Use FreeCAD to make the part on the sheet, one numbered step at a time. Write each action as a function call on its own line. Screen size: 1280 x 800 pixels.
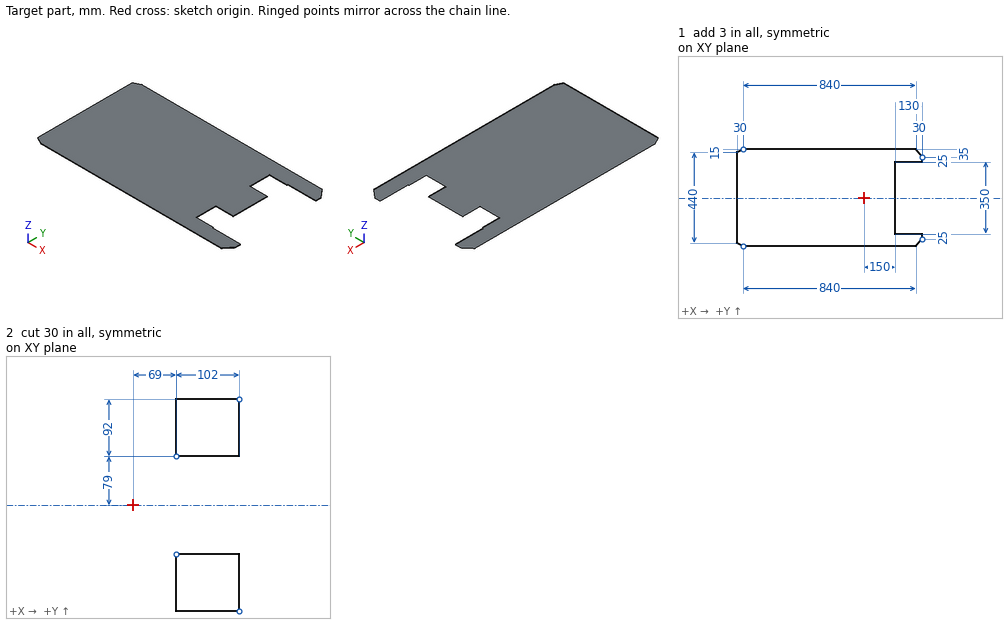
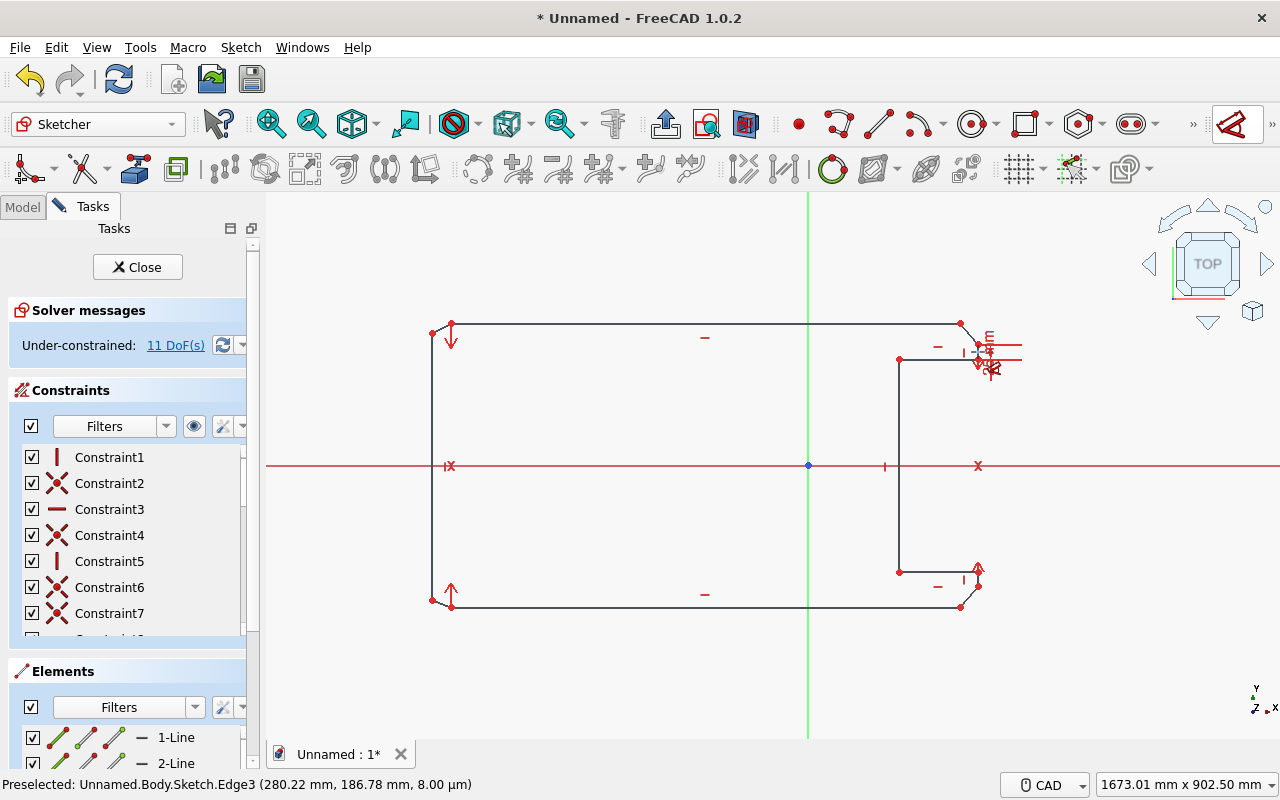
scroll(978, 583, up, 6)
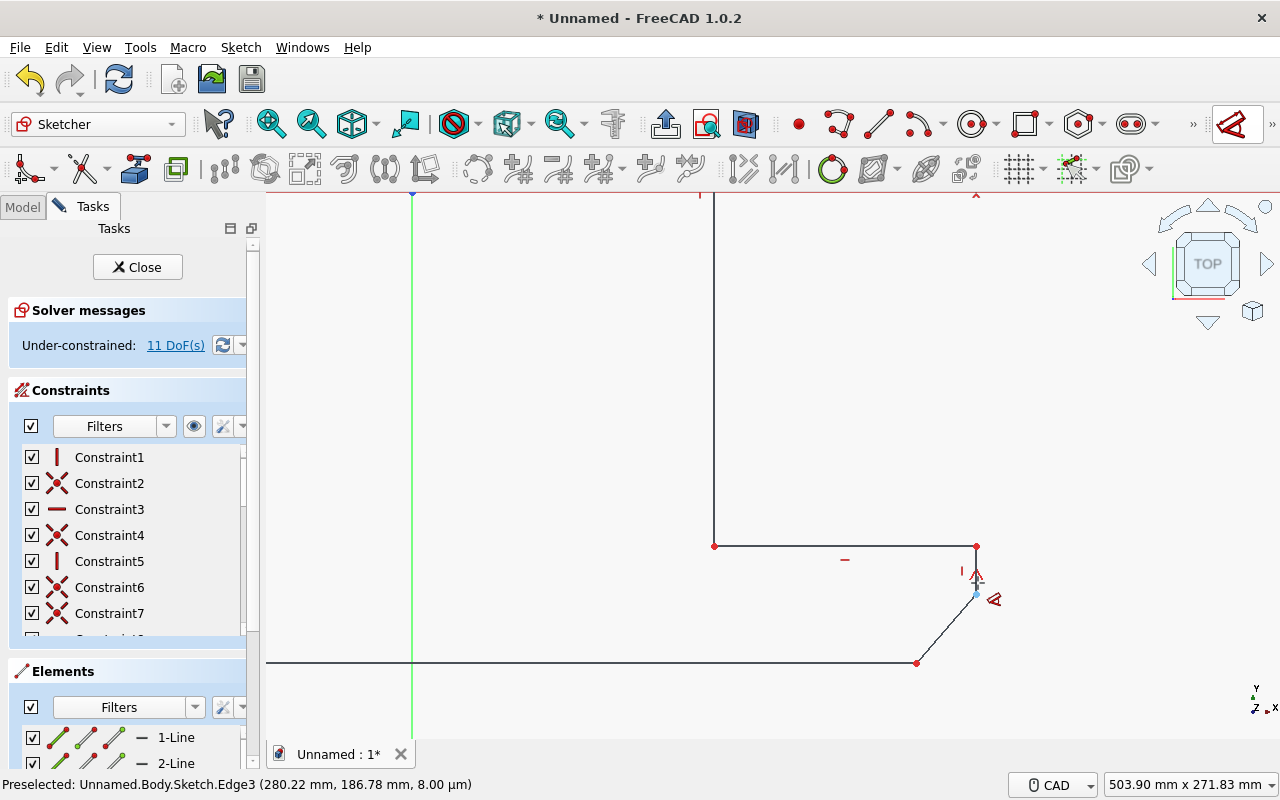
click(976, 580)
click(1010, 570)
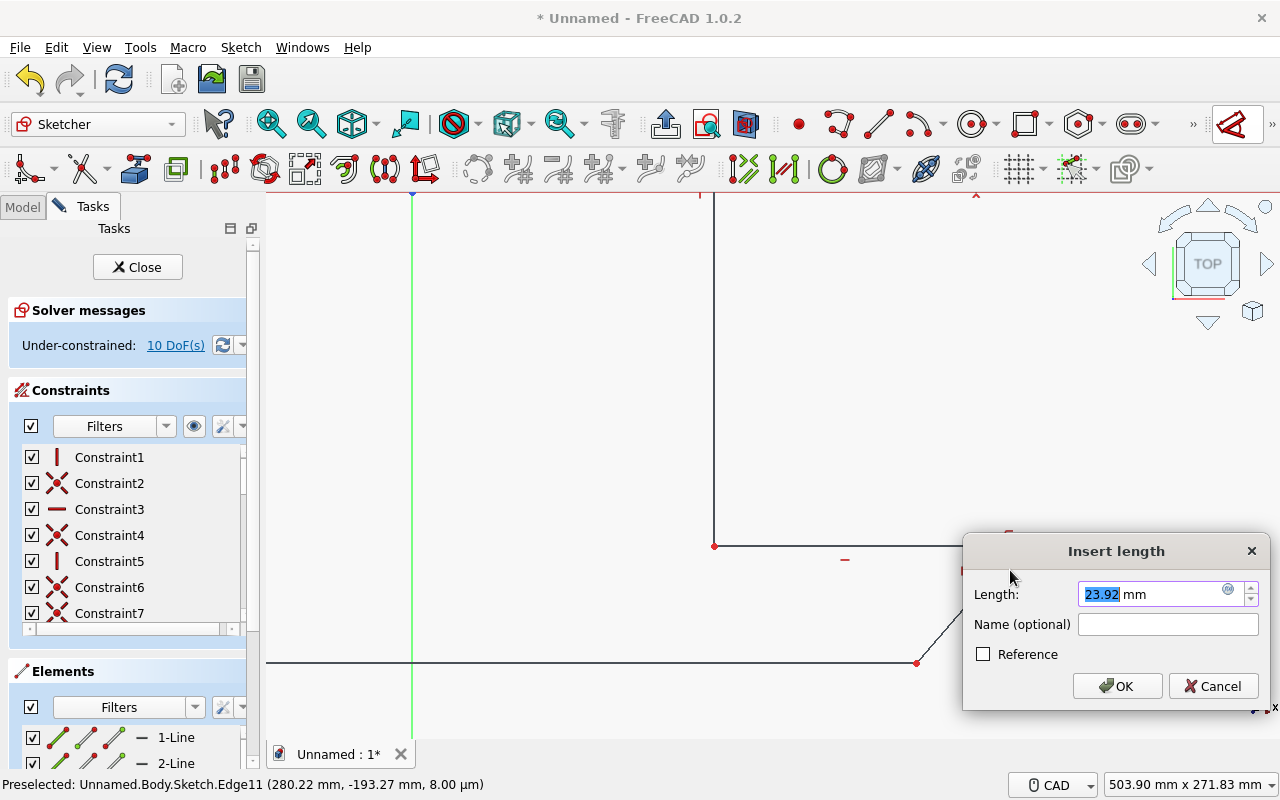
text(25)
key(Return)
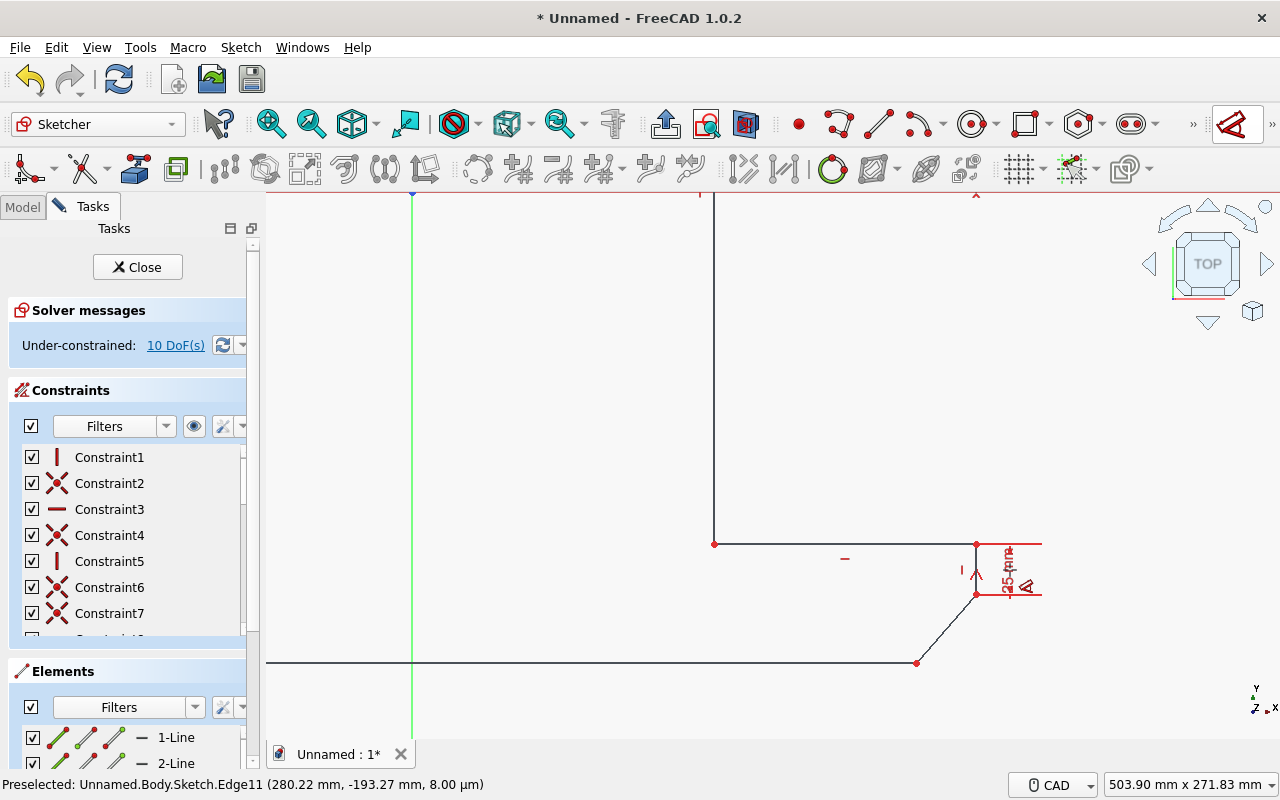
click(714, 333)
click(748, 382)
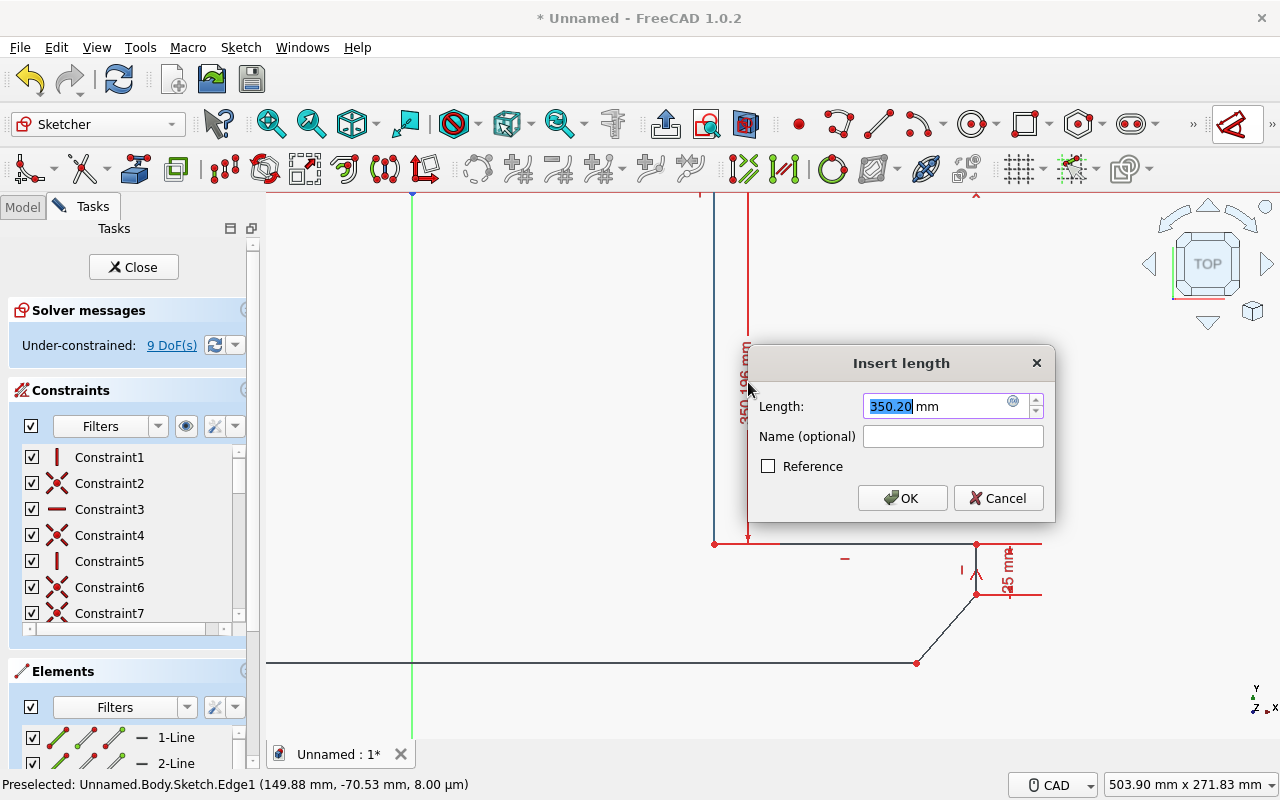
text(350)
key(Return)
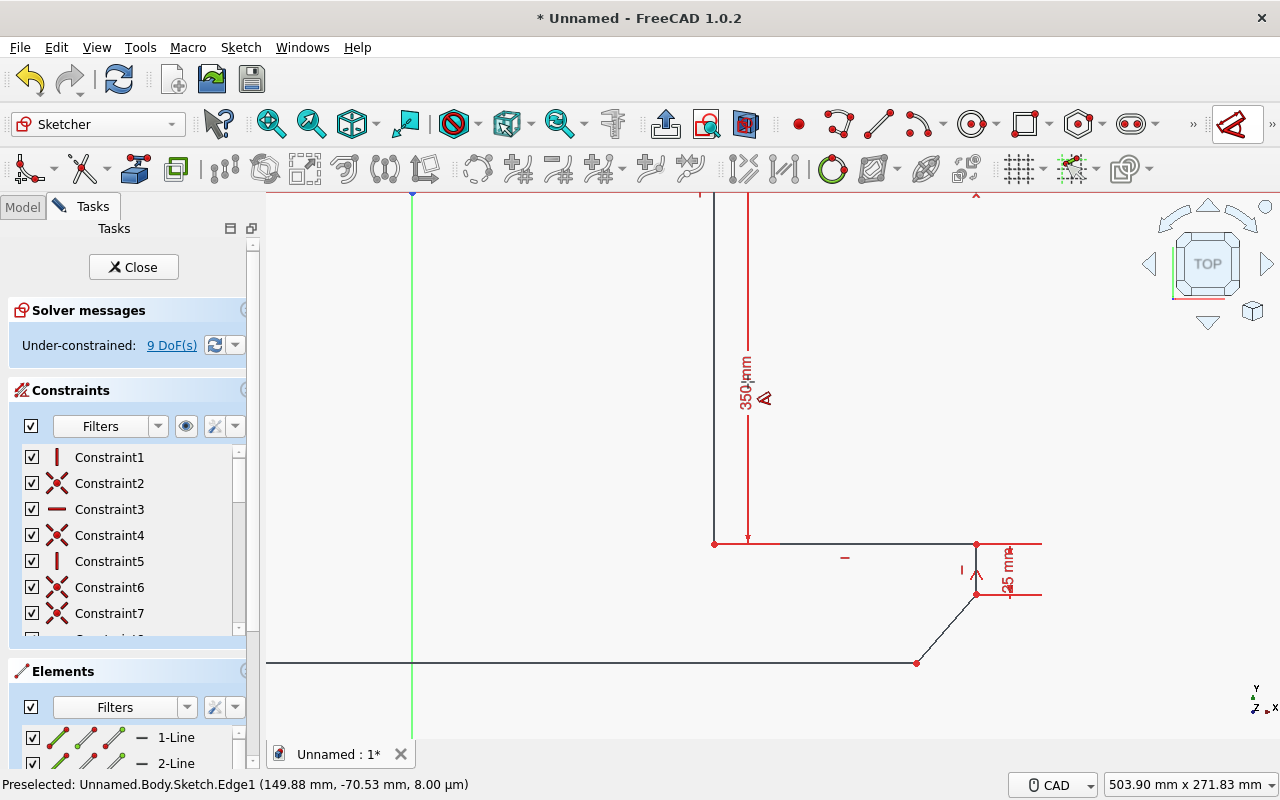
scroll(978, 583, down, 6)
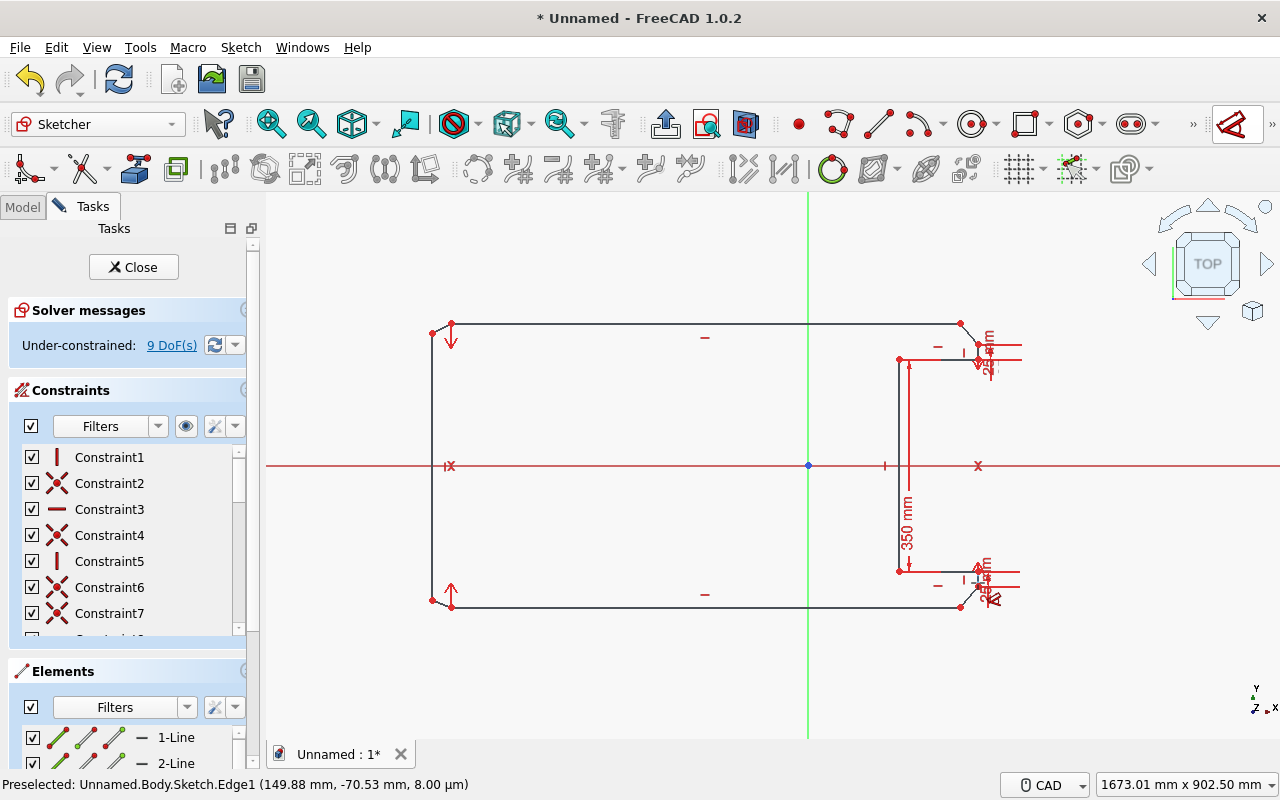
click(923, 360)
click(938, 394)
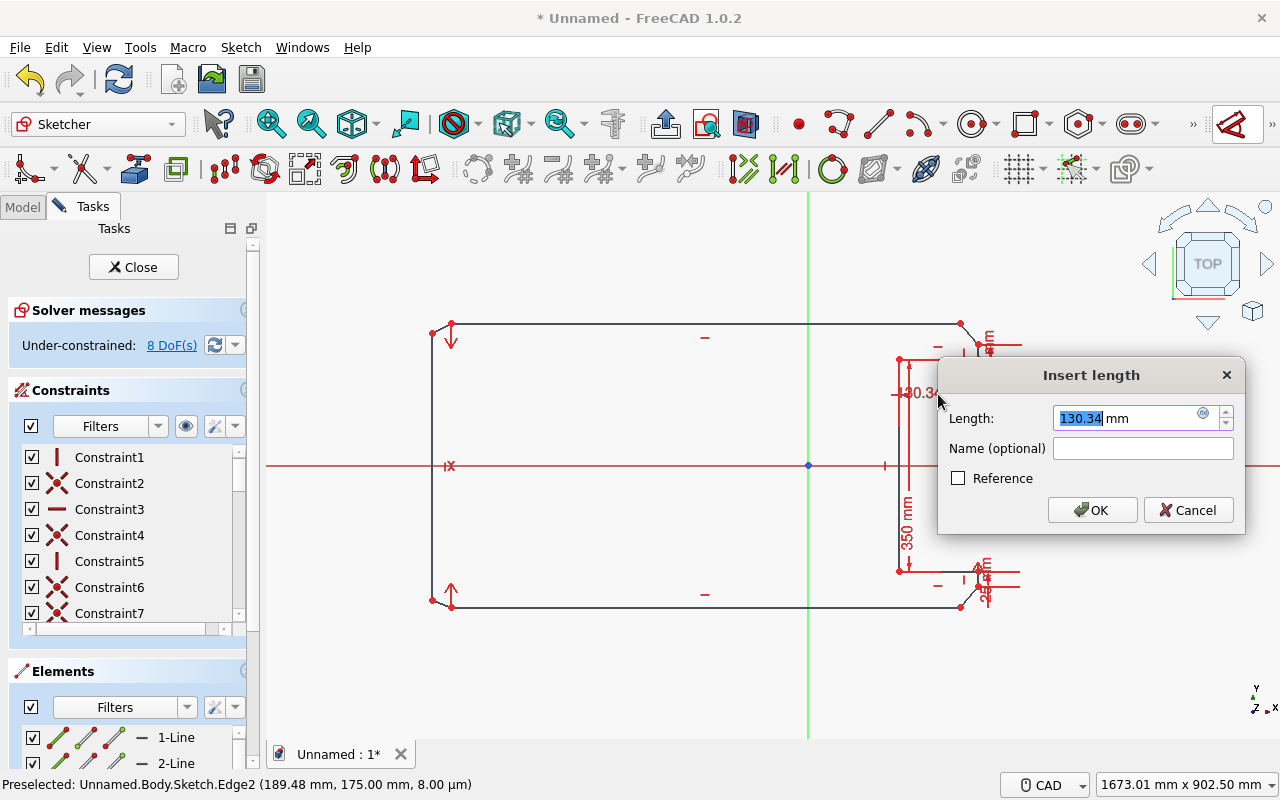
text(130)
key(Return)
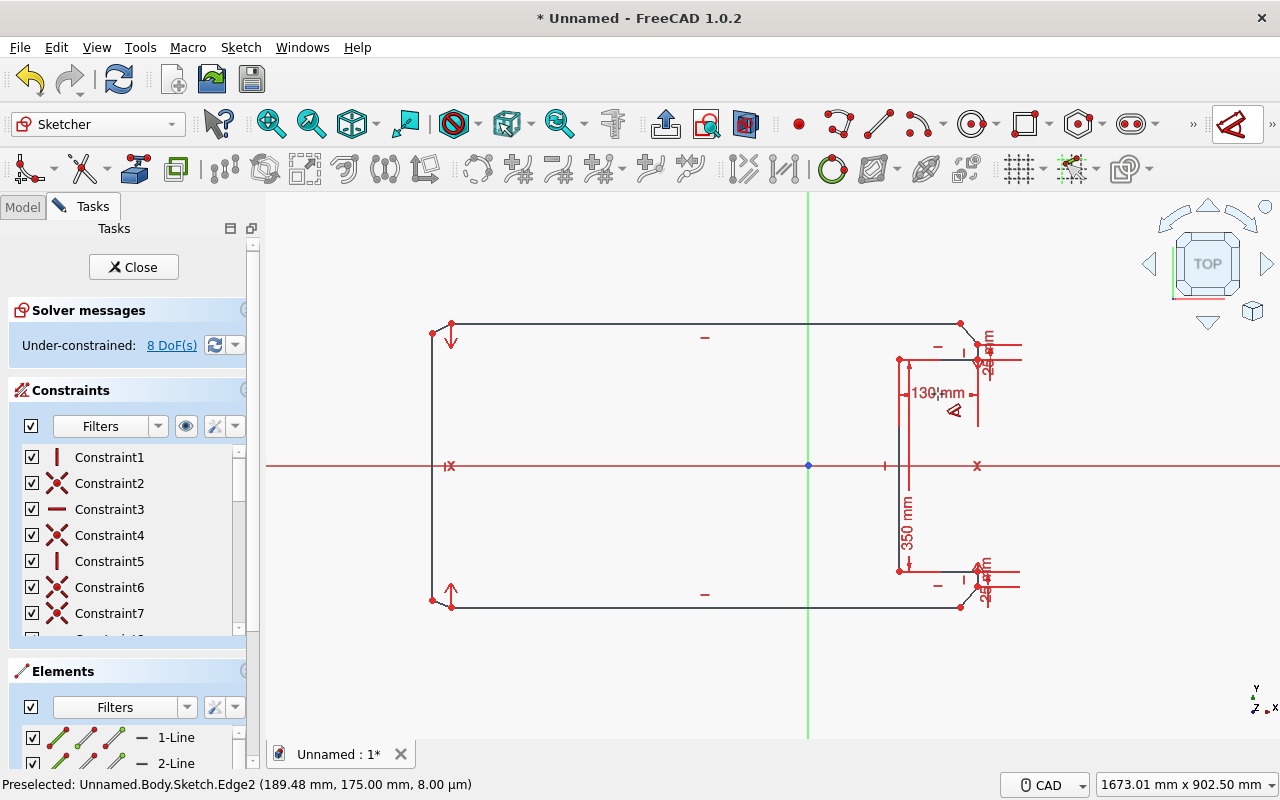
click(807, 324)
click(706, 290)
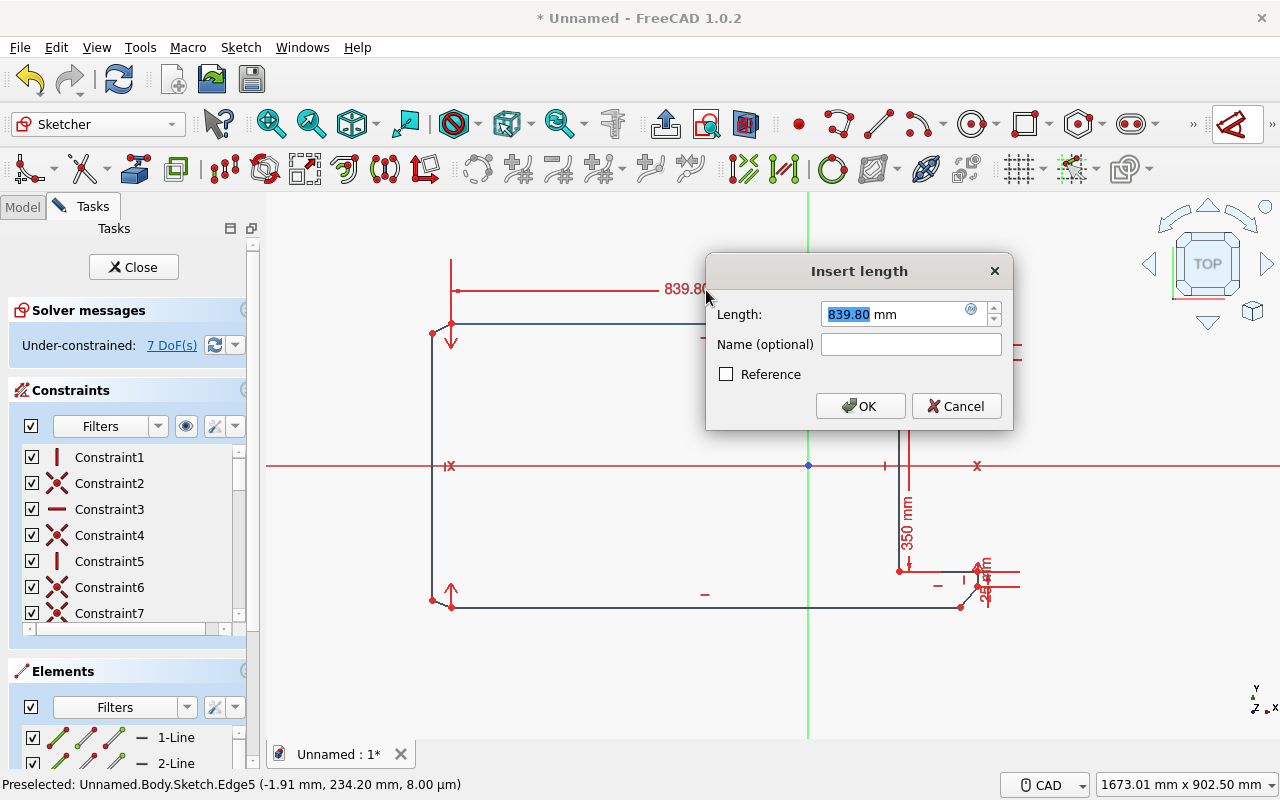
text(840)
key(Return)